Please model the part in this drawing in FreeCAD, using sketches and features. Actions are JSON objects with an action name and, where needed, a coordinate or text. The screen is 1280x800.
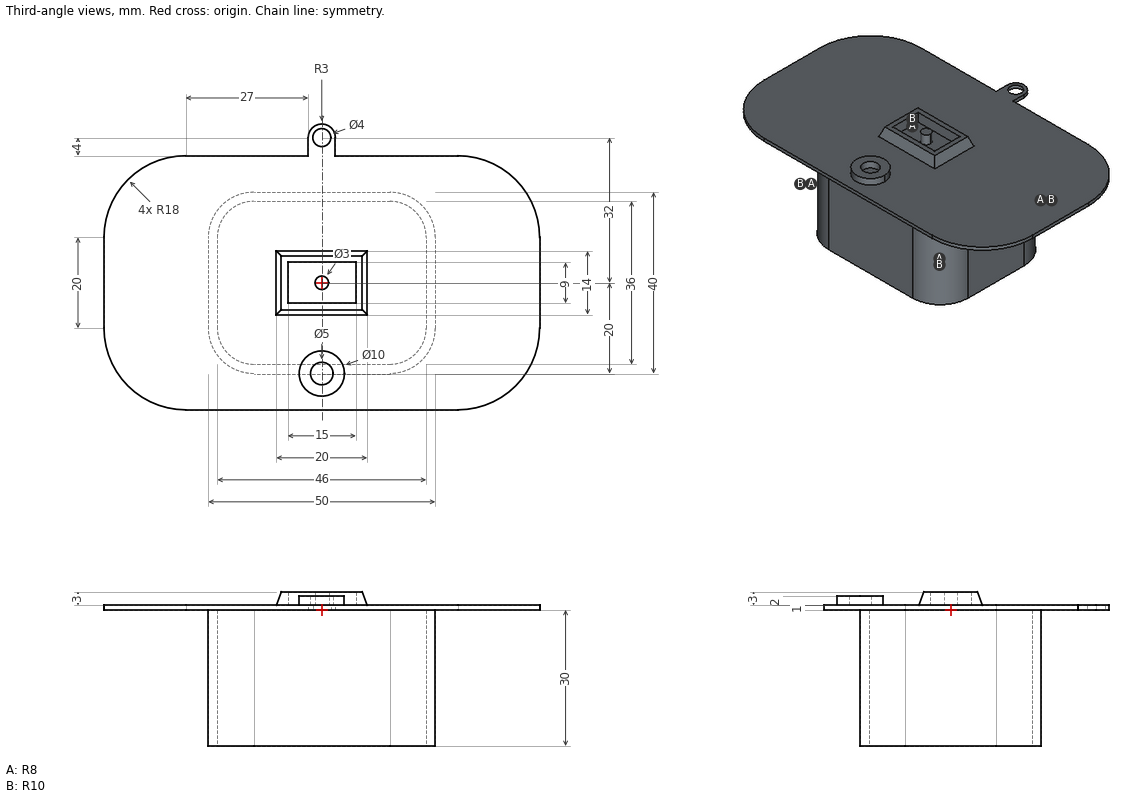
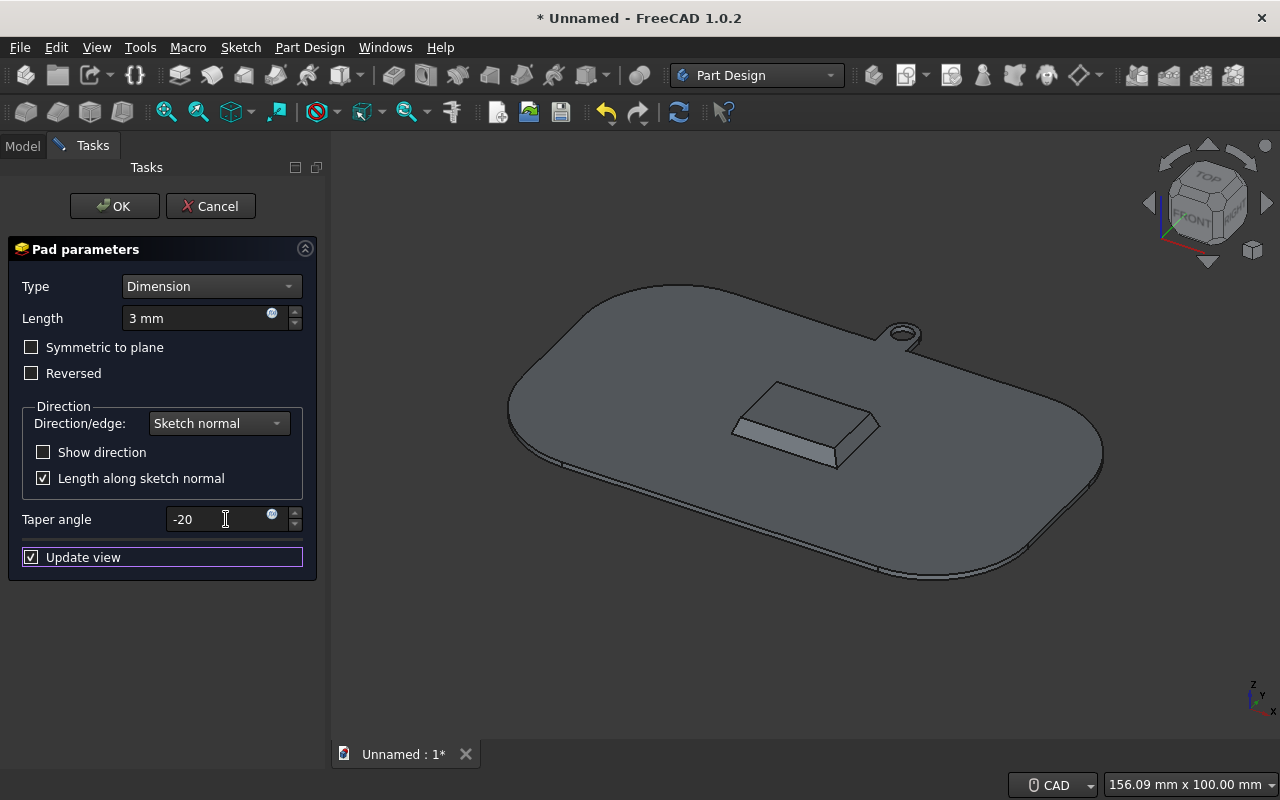
{"action": "left_click", "coordinate": [115, 206]}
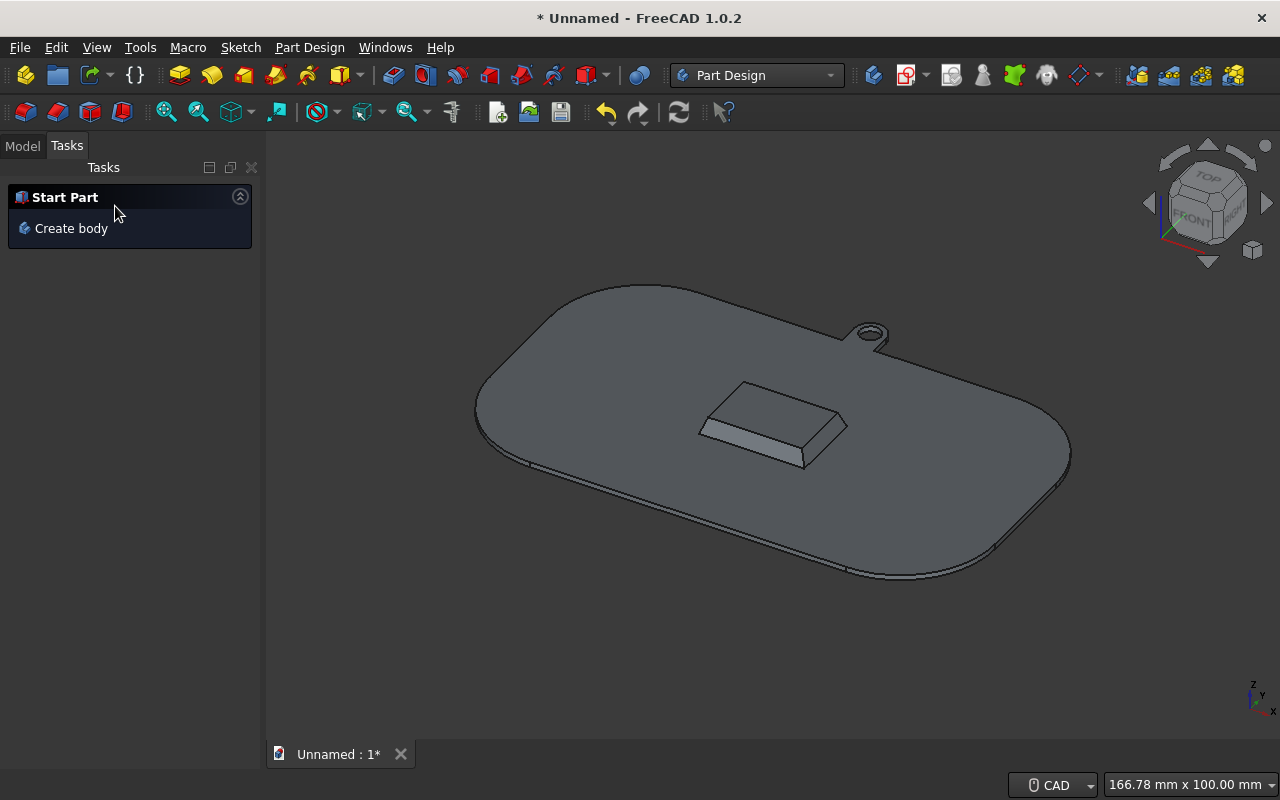
{"action": "left_click", "coordinate": [773, 414]}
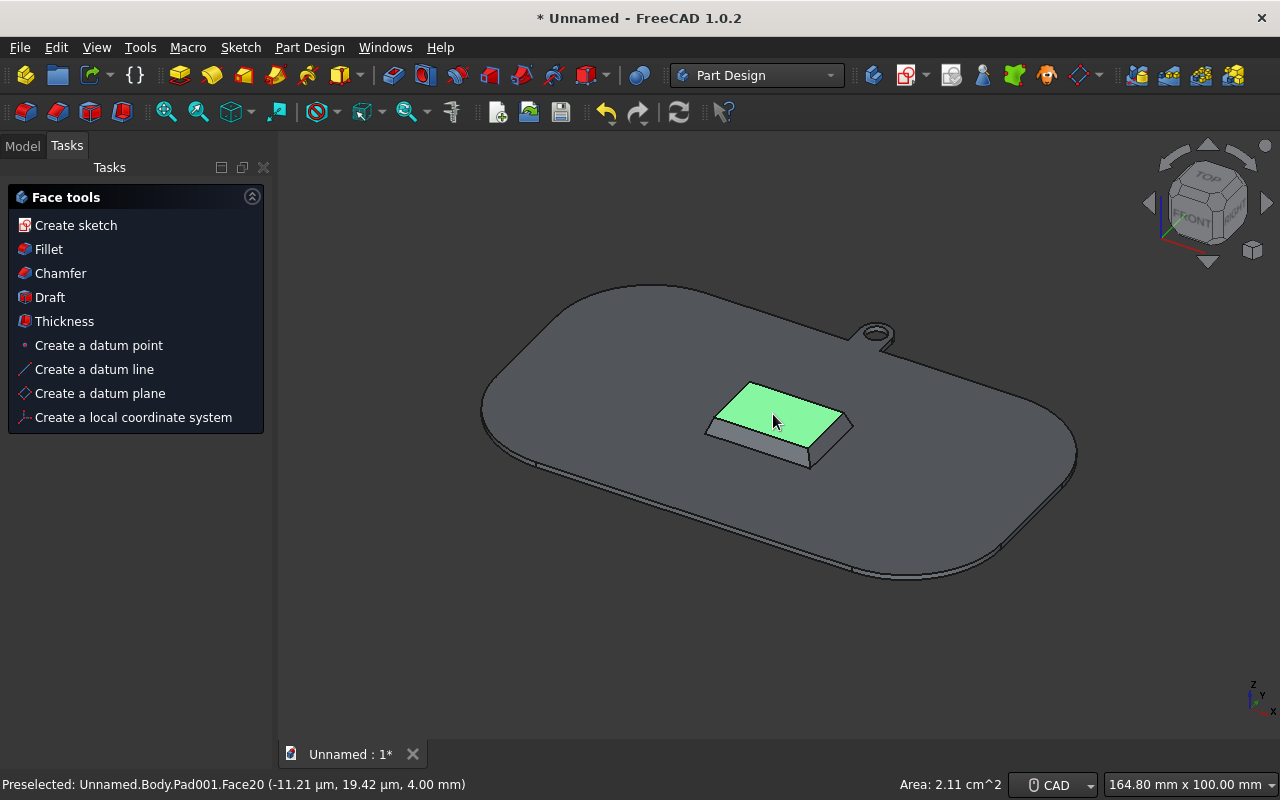
{"action": "left_click", "coordinate": [906, 76]}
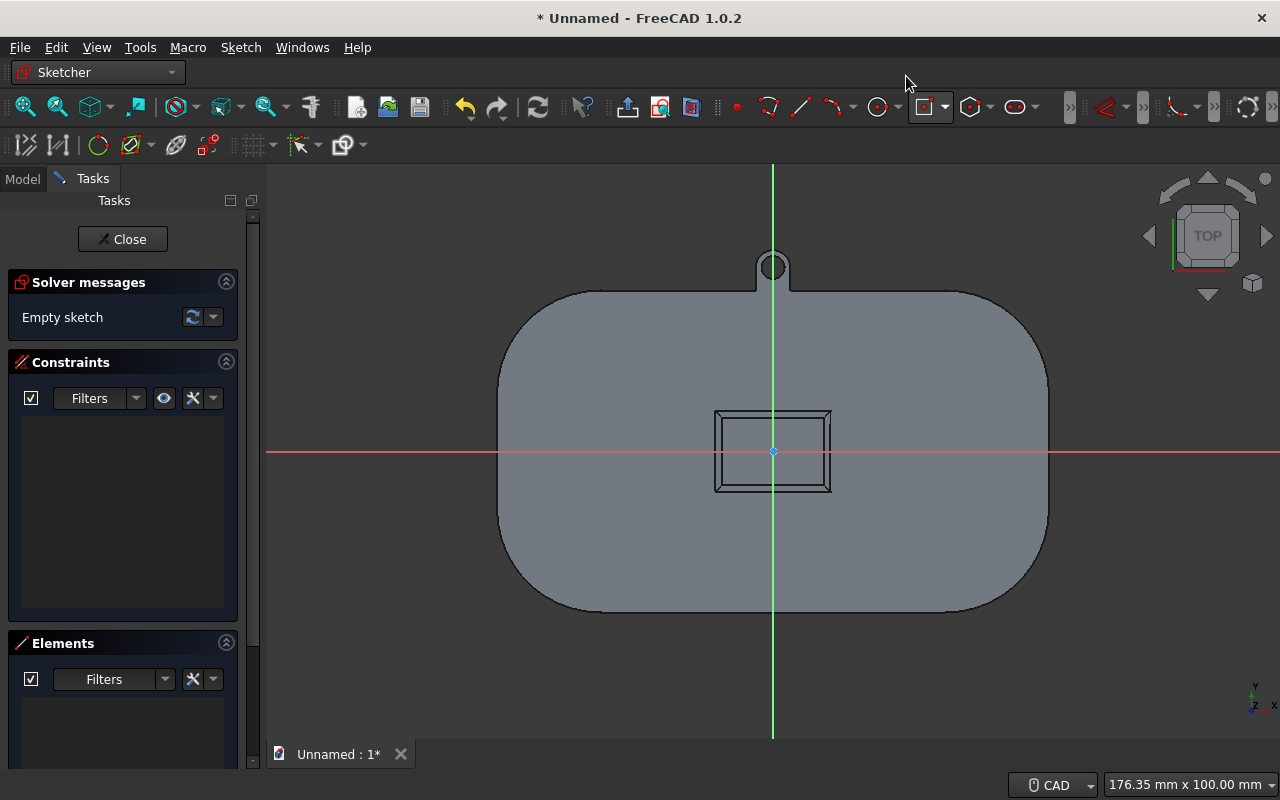
{"action": "scroll", "coordinate": [784, 452], "scroll_direction": "up", "scroll_amount": 10}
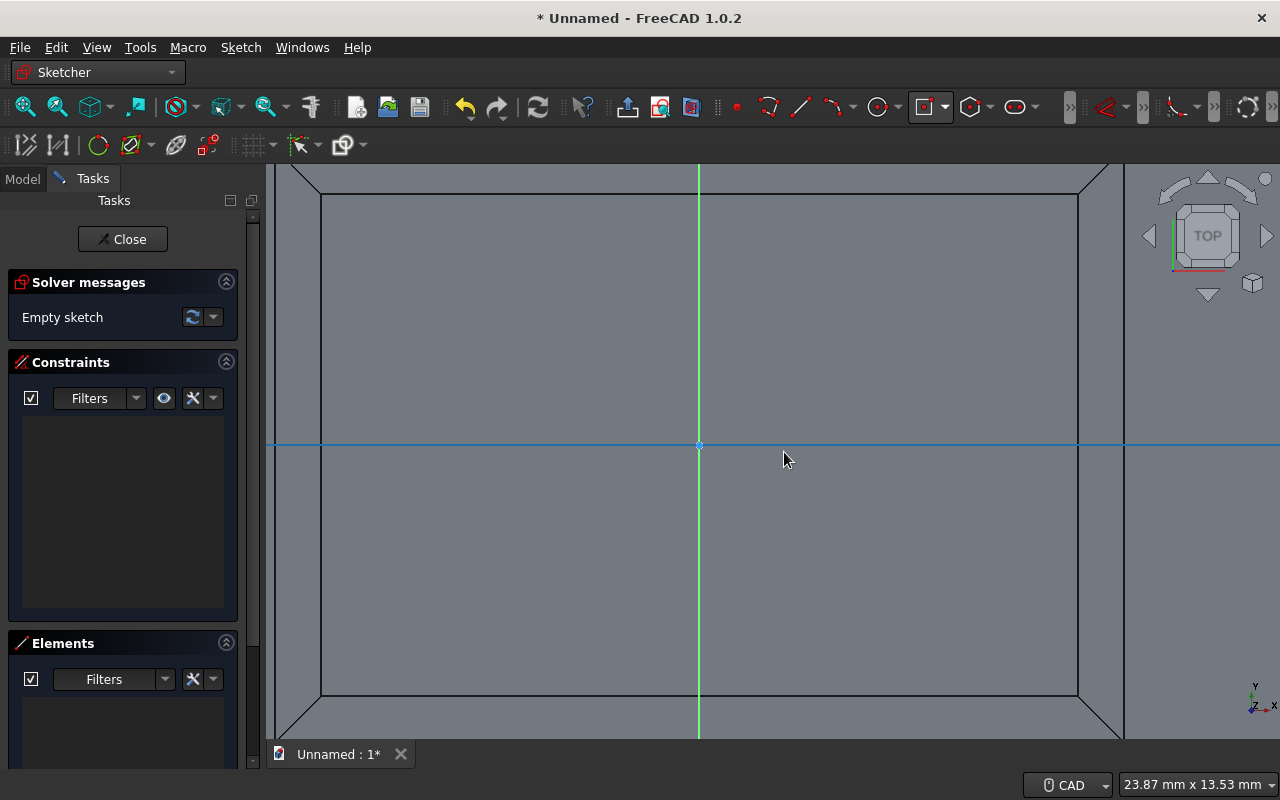
{"action": "left_click", "coordinate": [924, 108]}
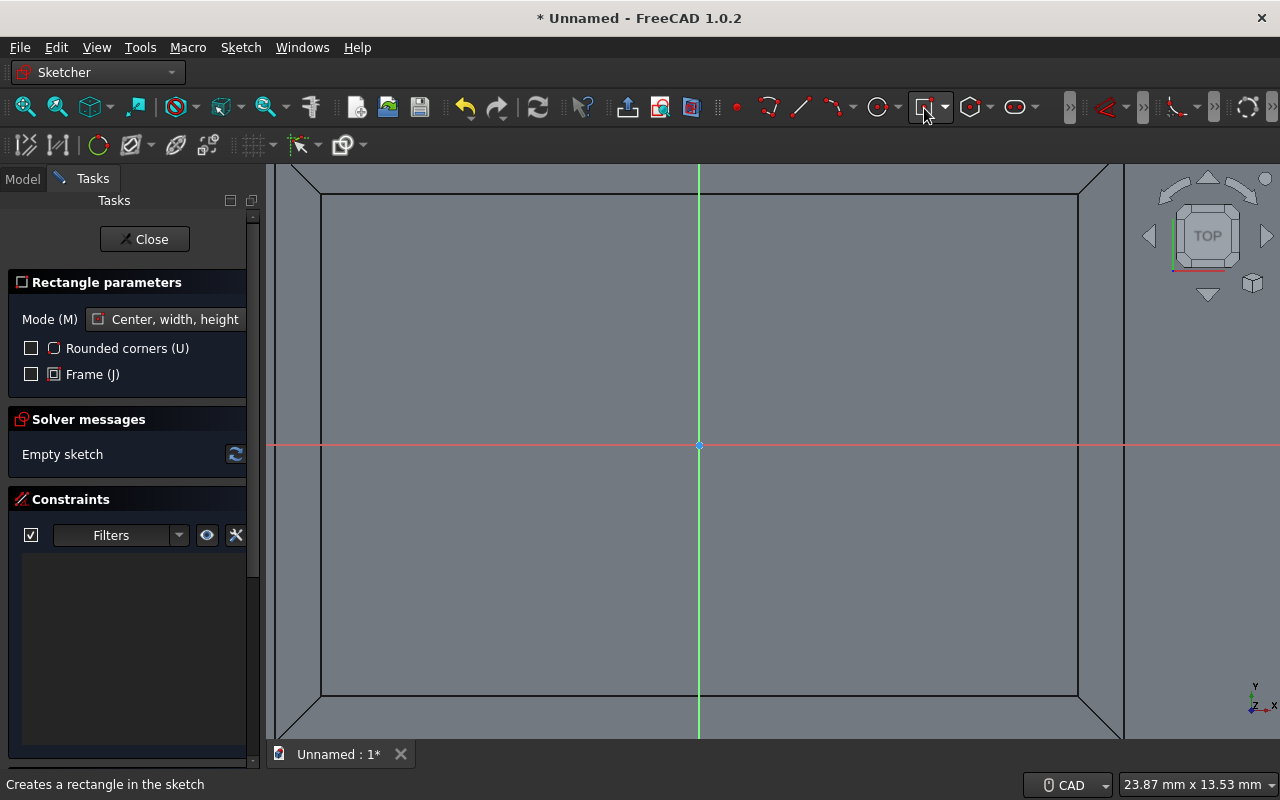
{"action": "left_click", "coordinate": [699, 445]}
{"action": "mouse_move", "coordinate": [1018, 254]}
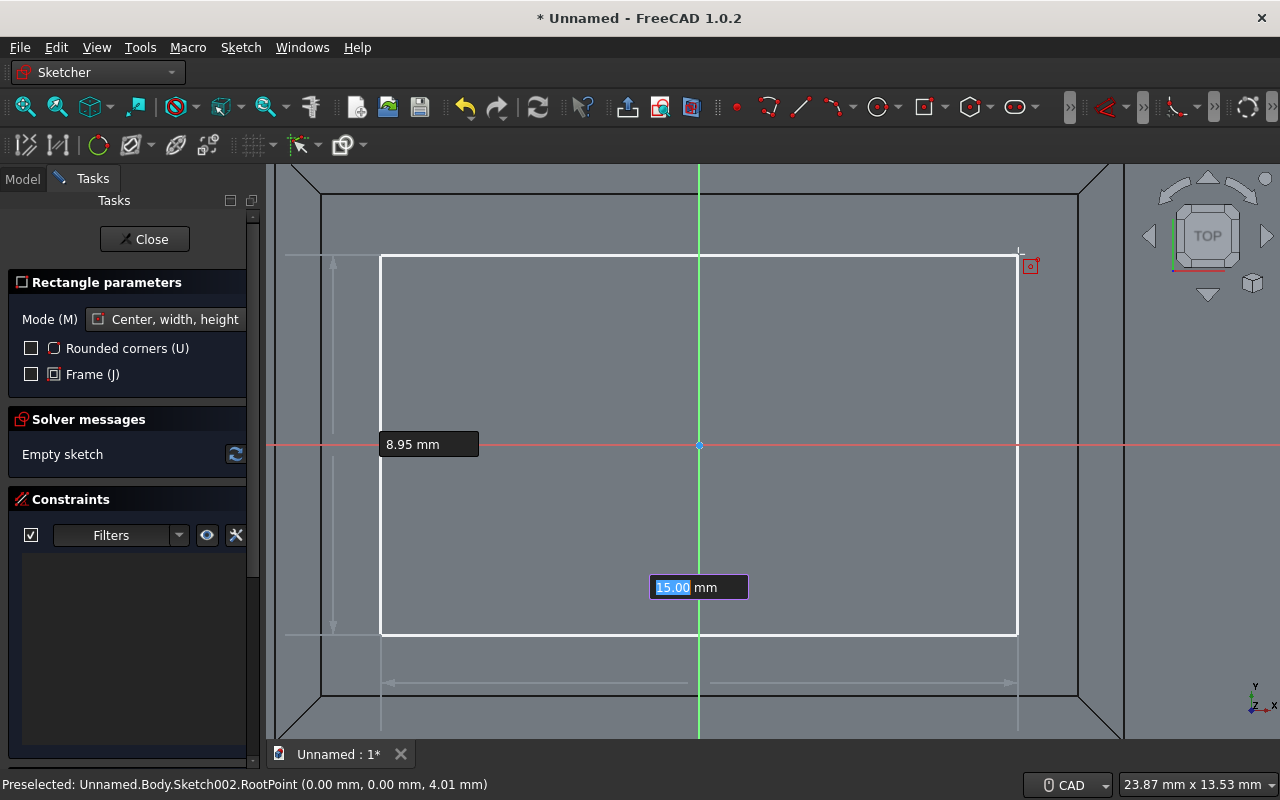
{"action": "type", "text": "15"}
{"action": "key", "text": "Tab"}
{"action": "type", "text": "9"}
{"action": "key", "text": "Return"}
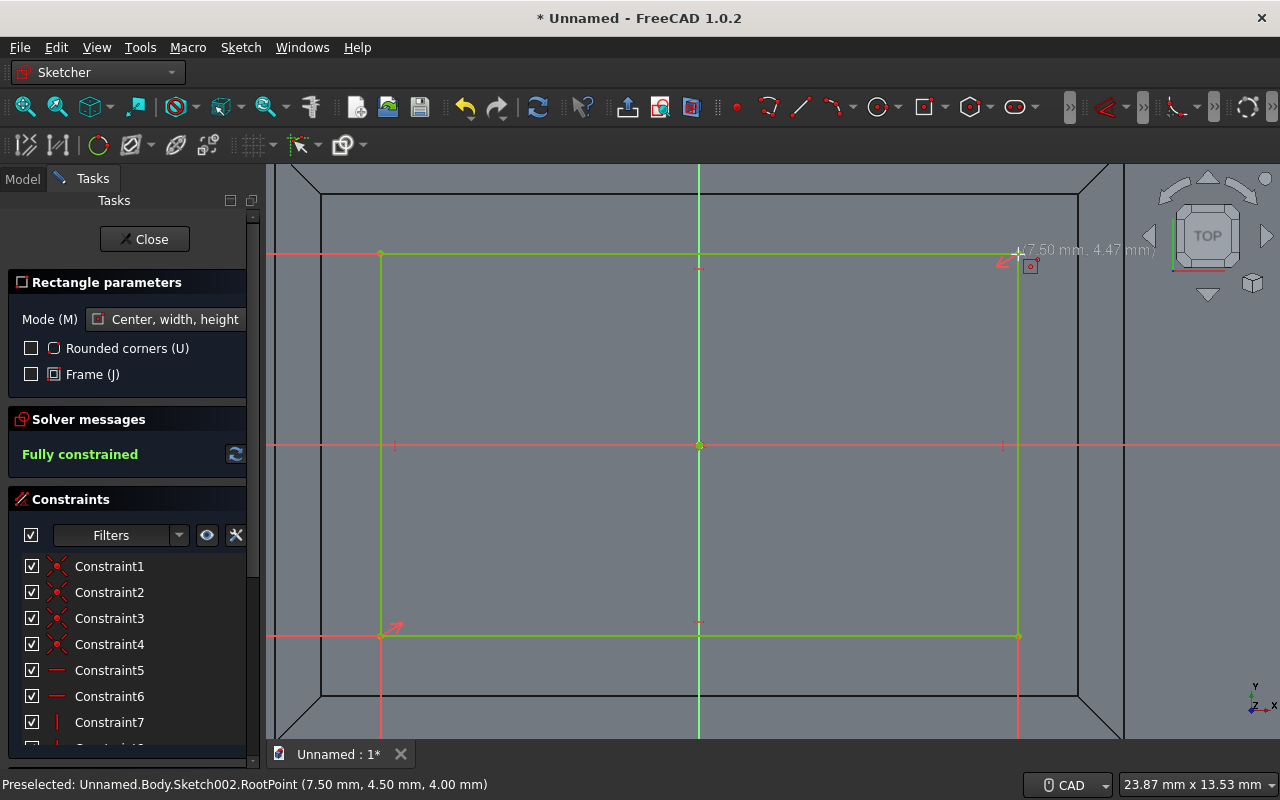
{"action": "left_click", "coordinate": [878, 108]}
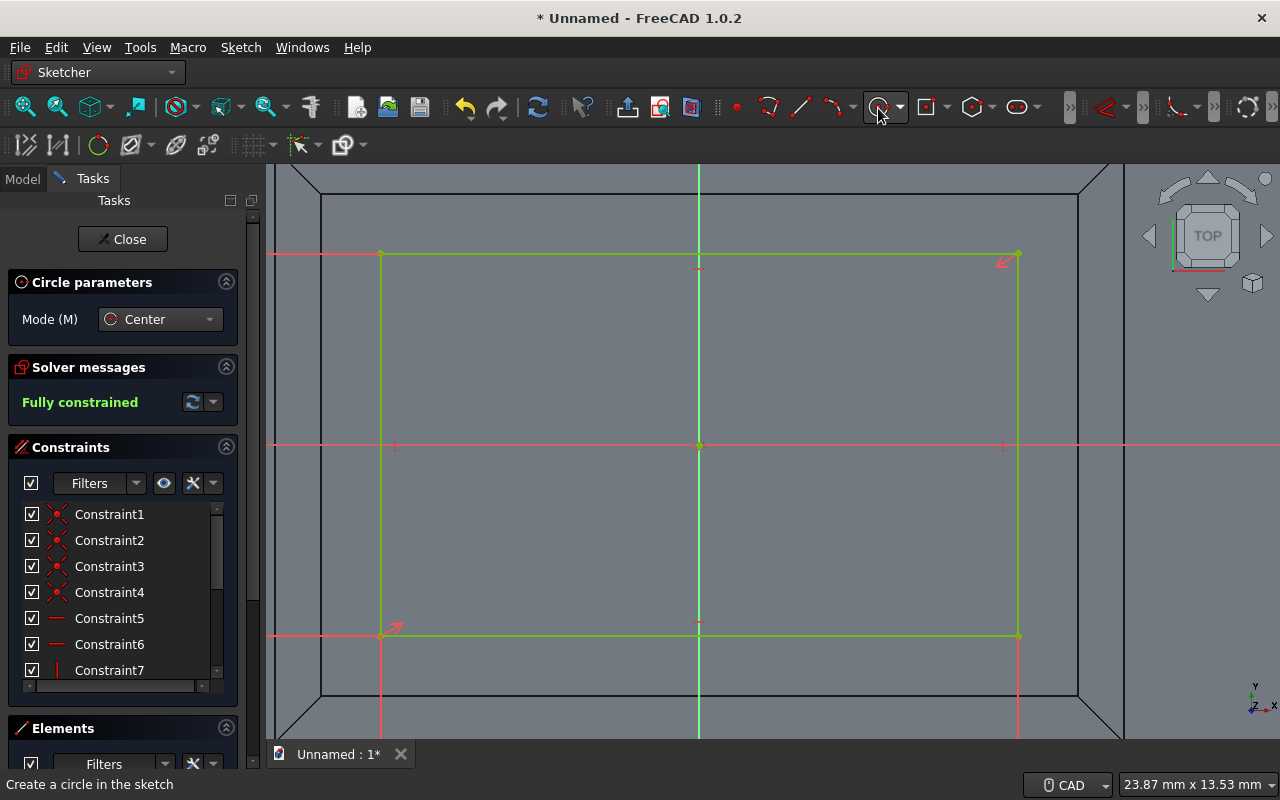
{"action": "left_click", "coordinate": [699, 445]}
{"action": "mouse_move", "coordinate": [745, 400]}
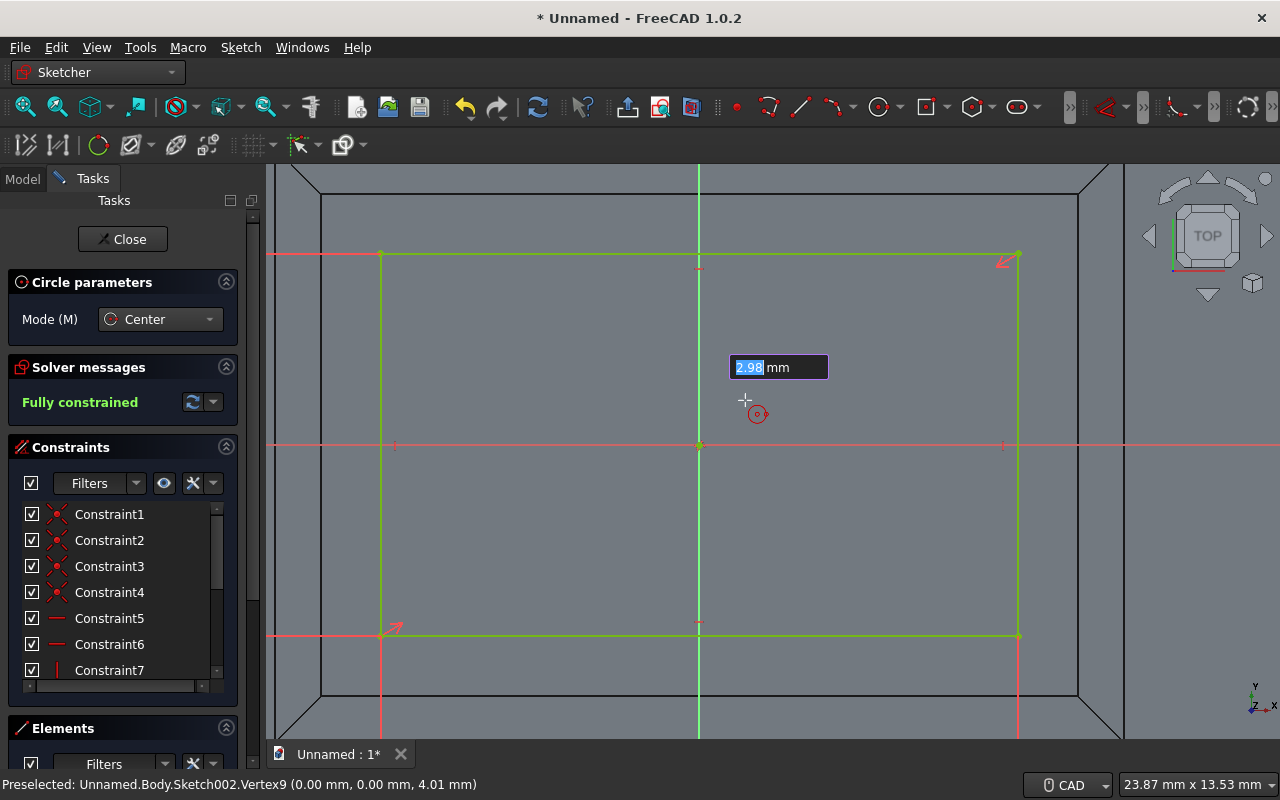
{"action": "type", "text": "3"}
{"action": "key", "text": "Return"}
{"action": "key", "text": "Escape"}